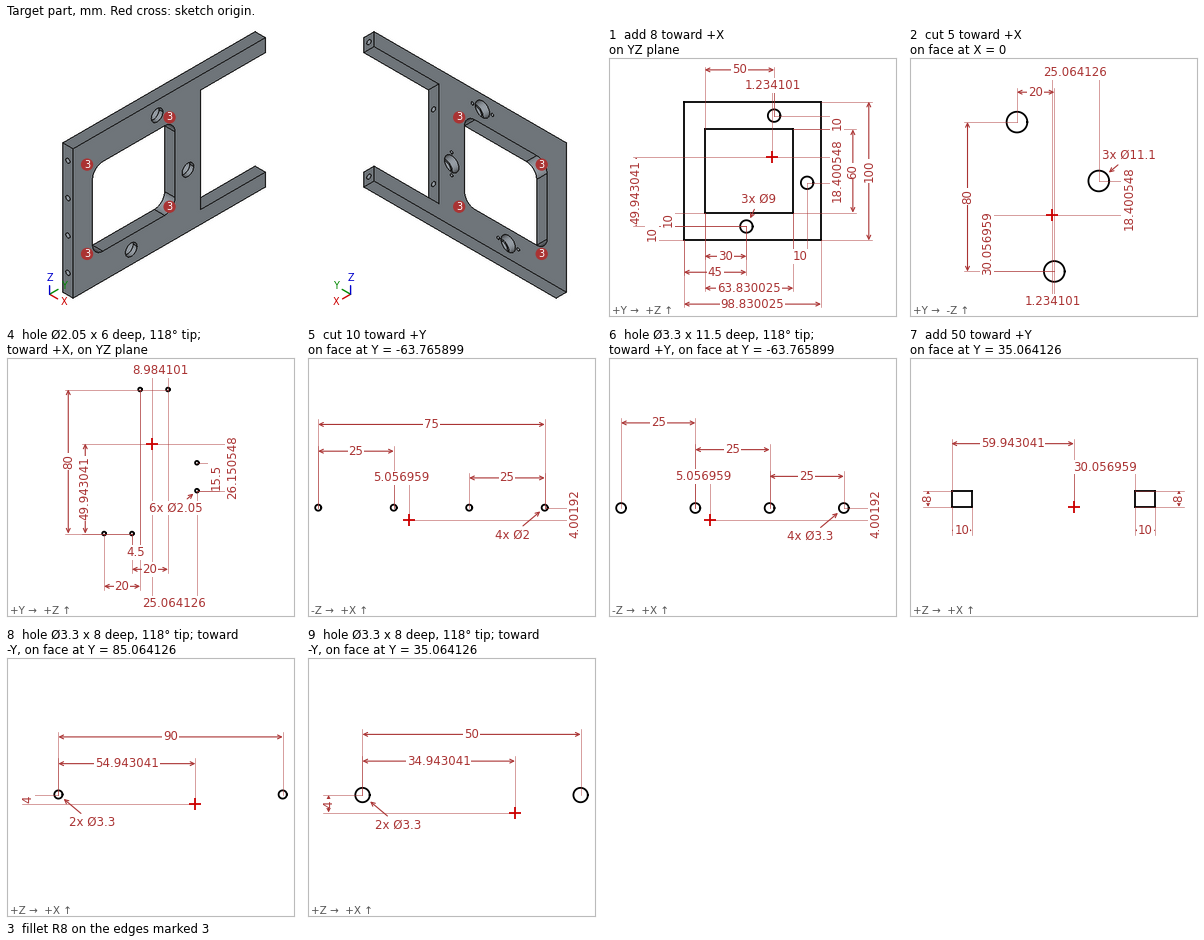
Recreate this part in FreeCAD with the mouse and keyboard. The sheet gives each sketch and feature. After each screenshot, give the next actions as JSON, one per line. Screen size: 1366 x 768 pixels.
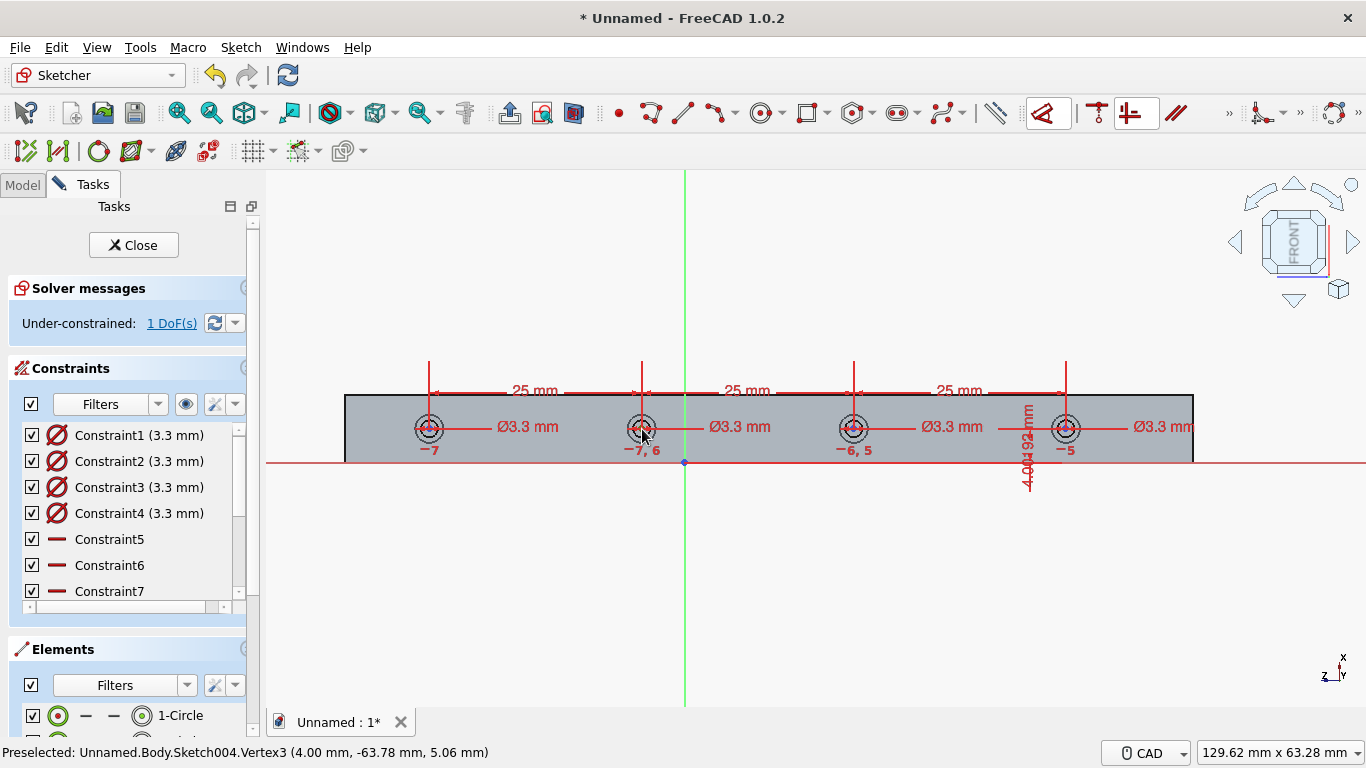
{"action": "left_click", "coordinate": [1066, 114]}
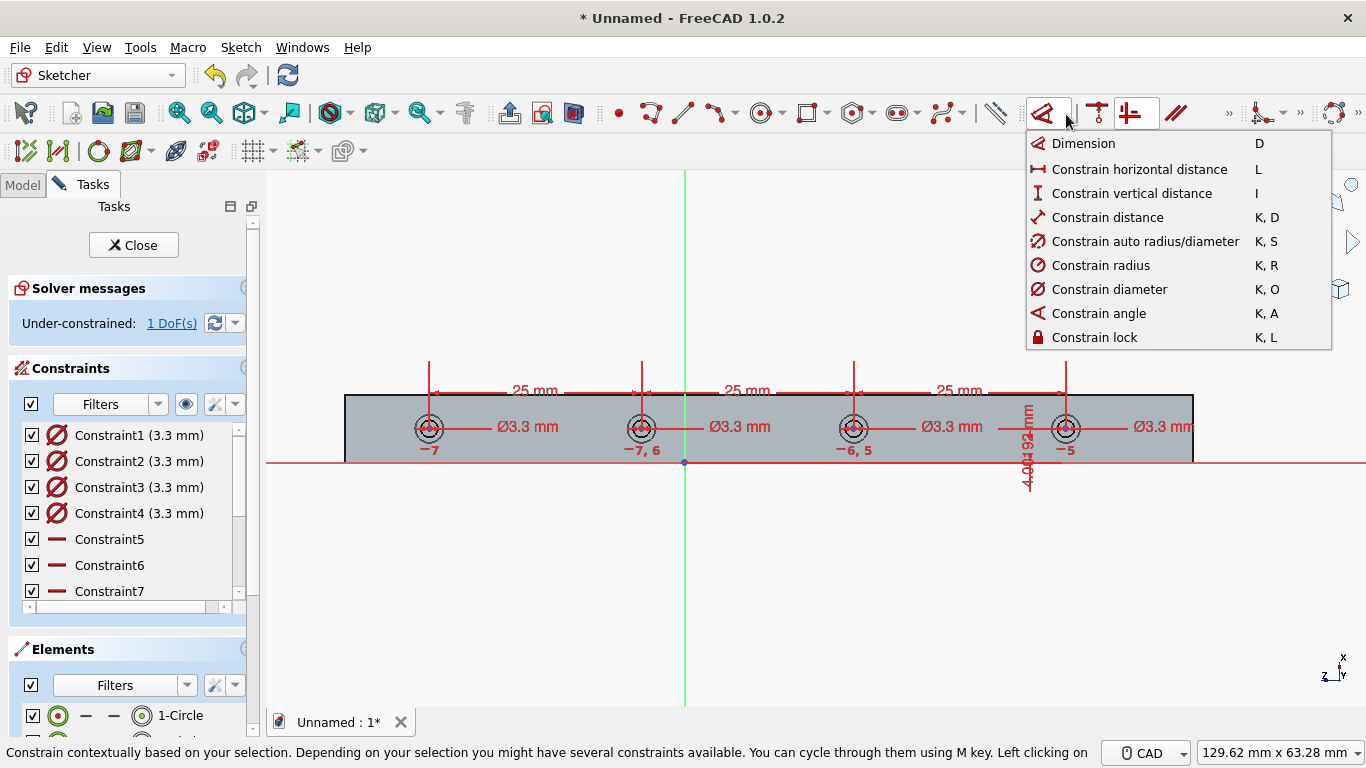
{"action": "left_click", "coordinate": [1179, 169]}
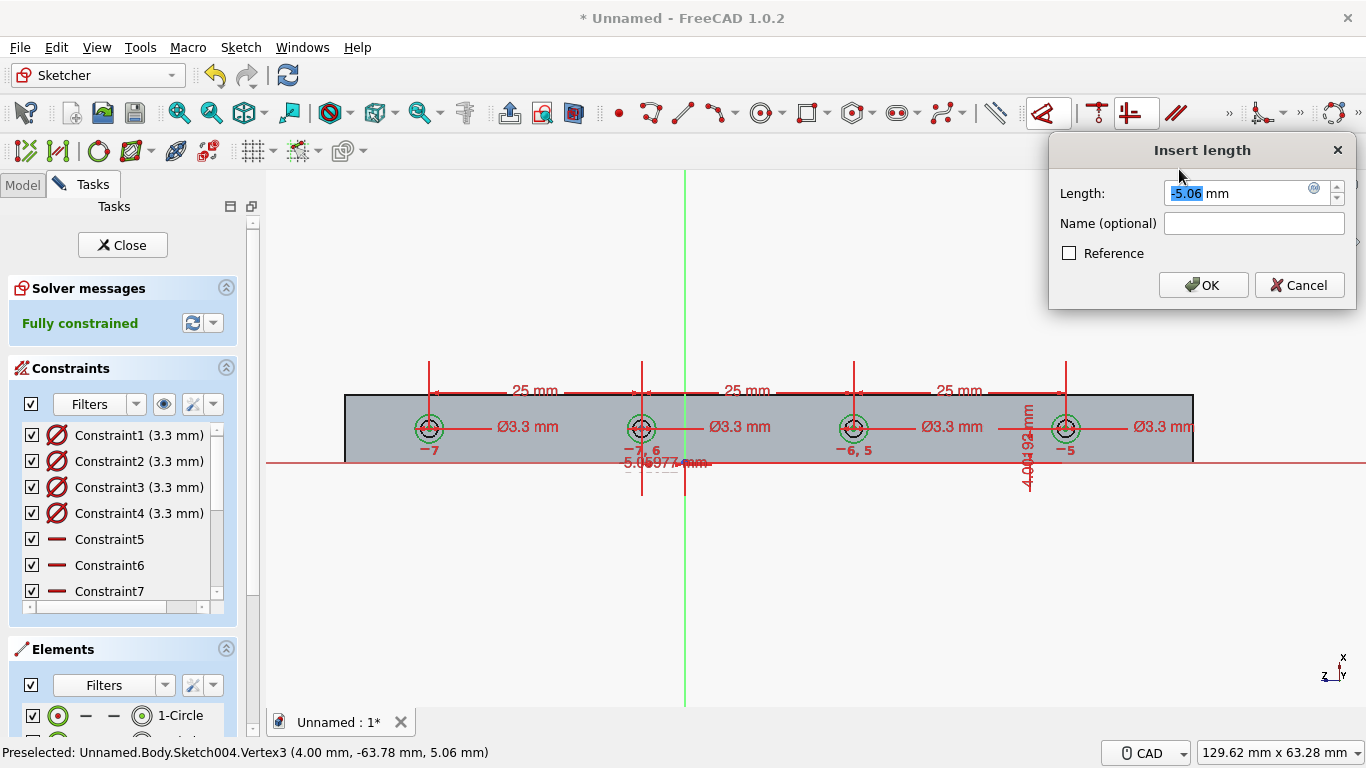
{"action": "type", "text": "-5.056959"}
{"action": "key", "text": "Return"}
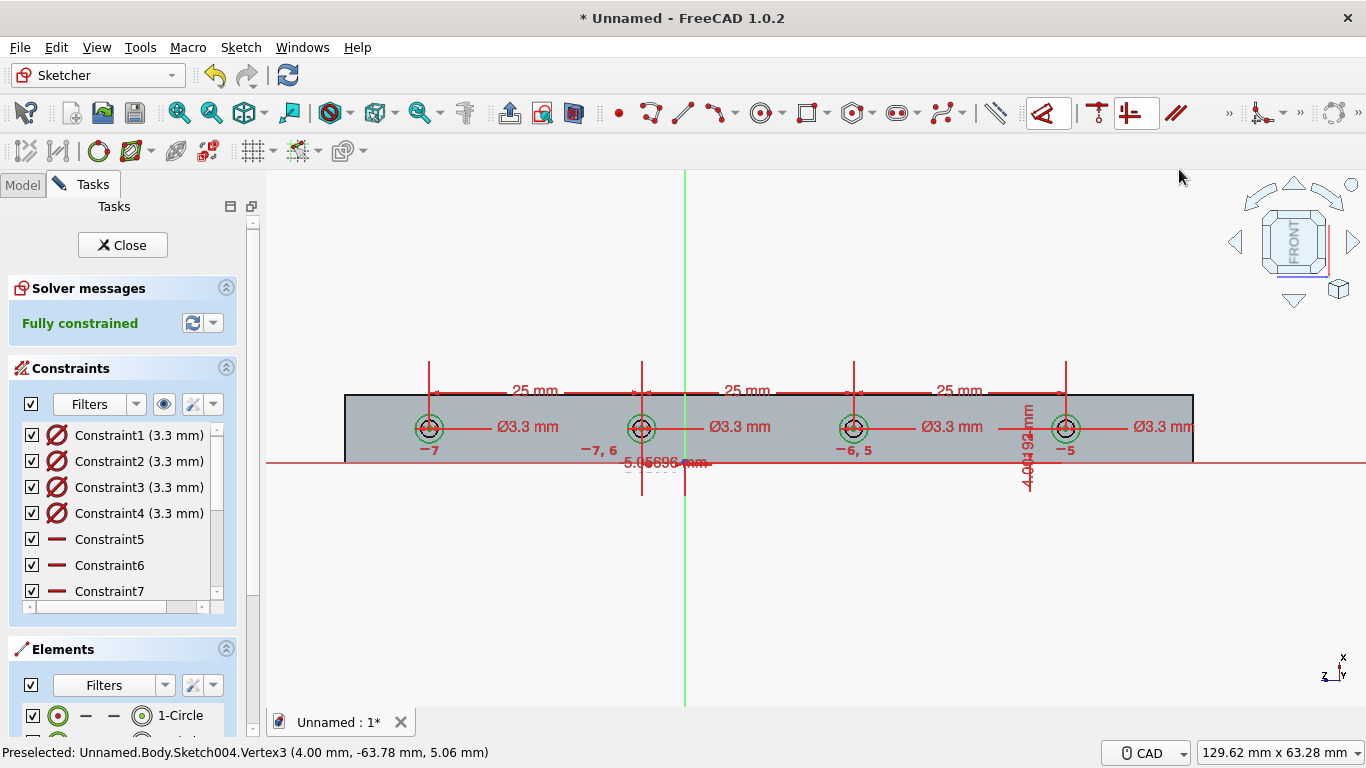
{"action": "left_click", "coordinate": [123, 245]}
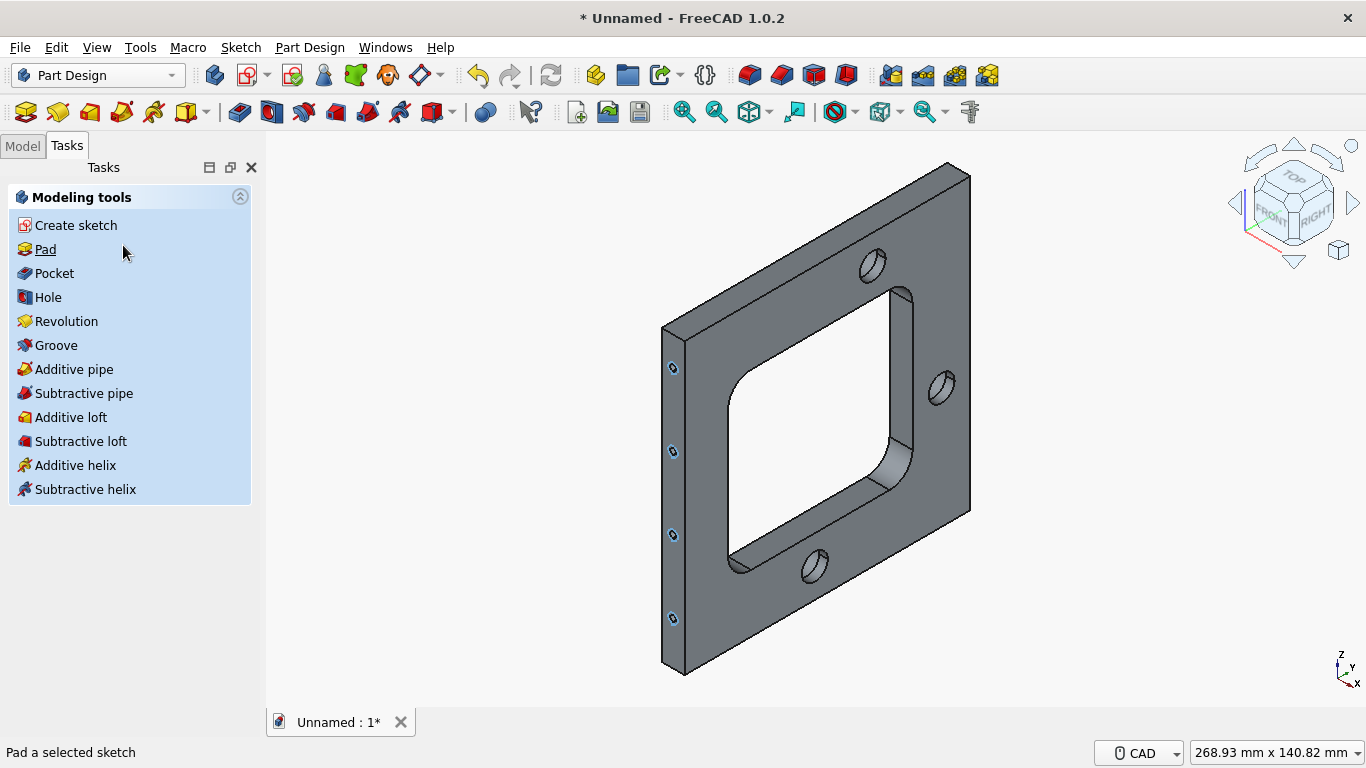
{"action": "left_click", "coordinate": [272, 112]}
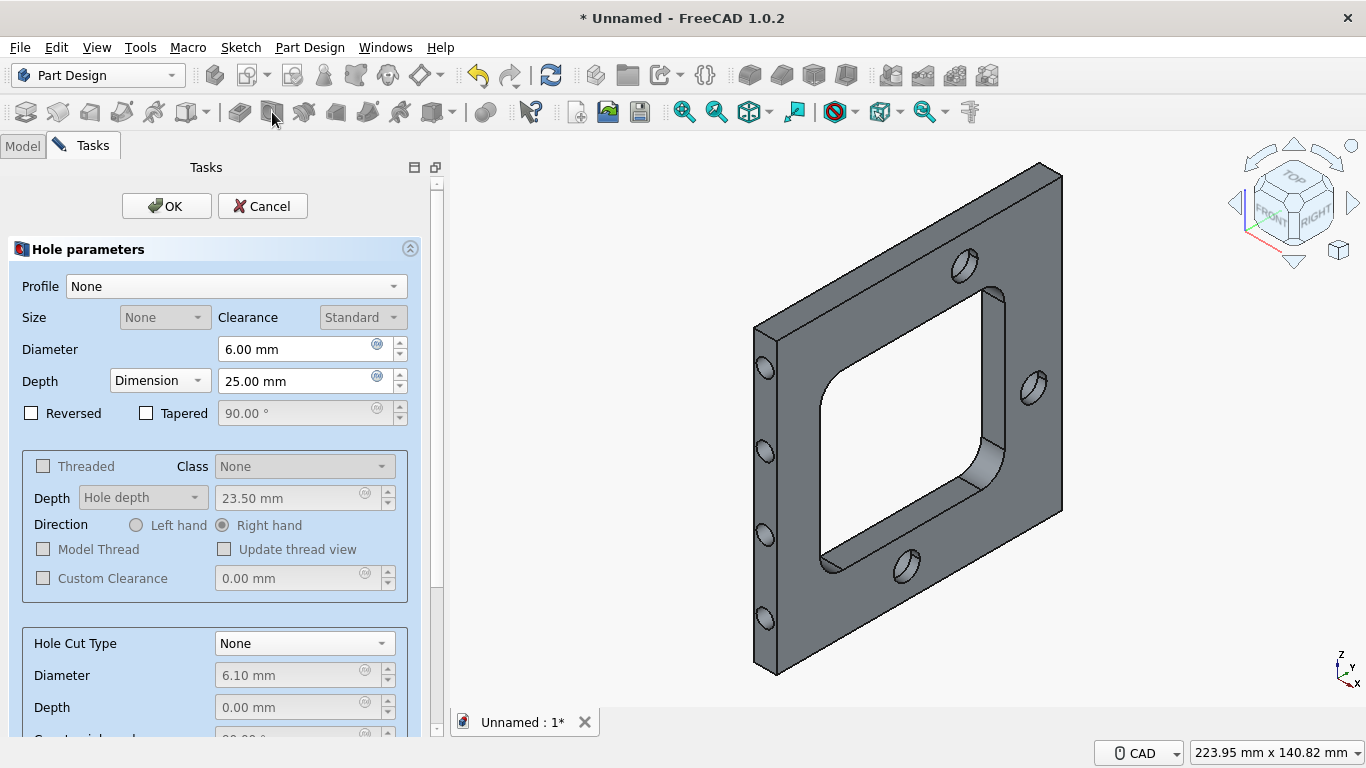
{"action": "triple_click", "coordinate": [305, 349]}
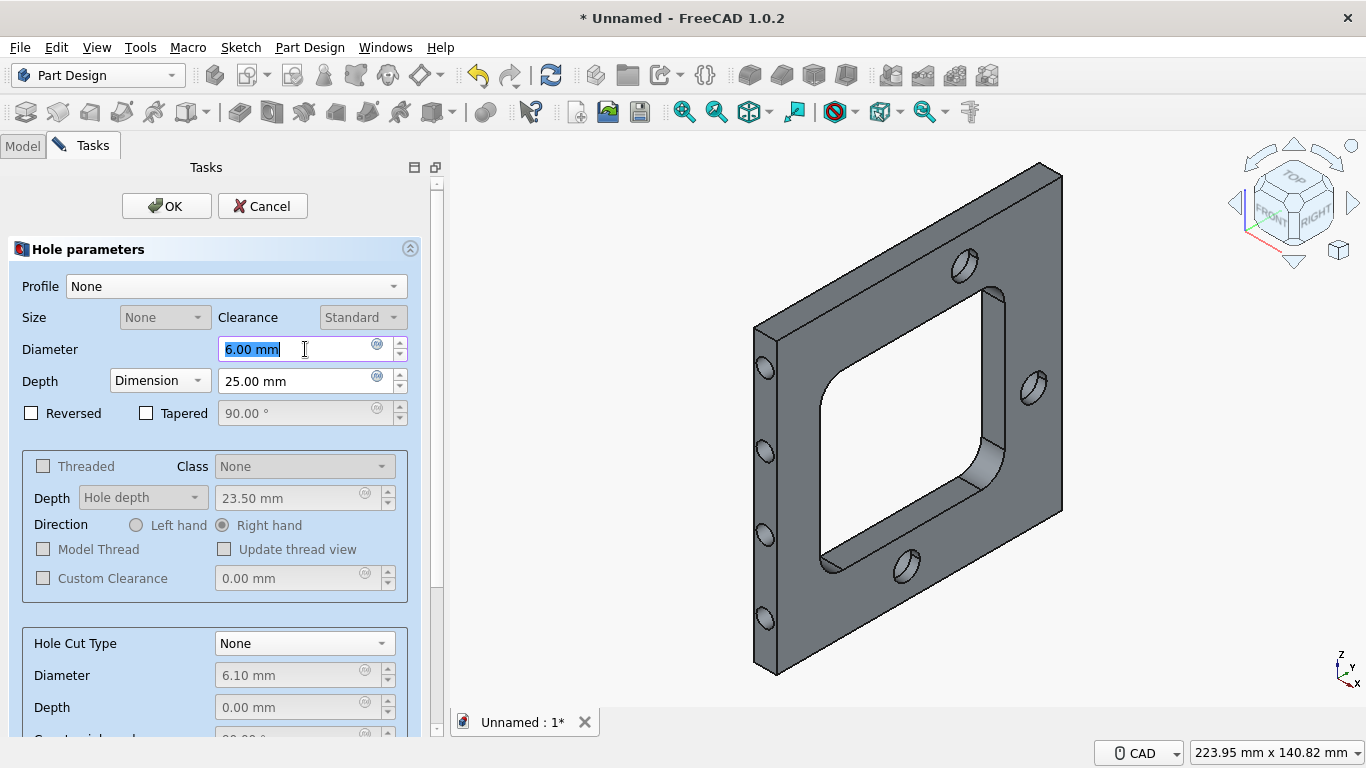
{"action": "type", "text": "3.3"}
{"action": "key", "text": "Tab"}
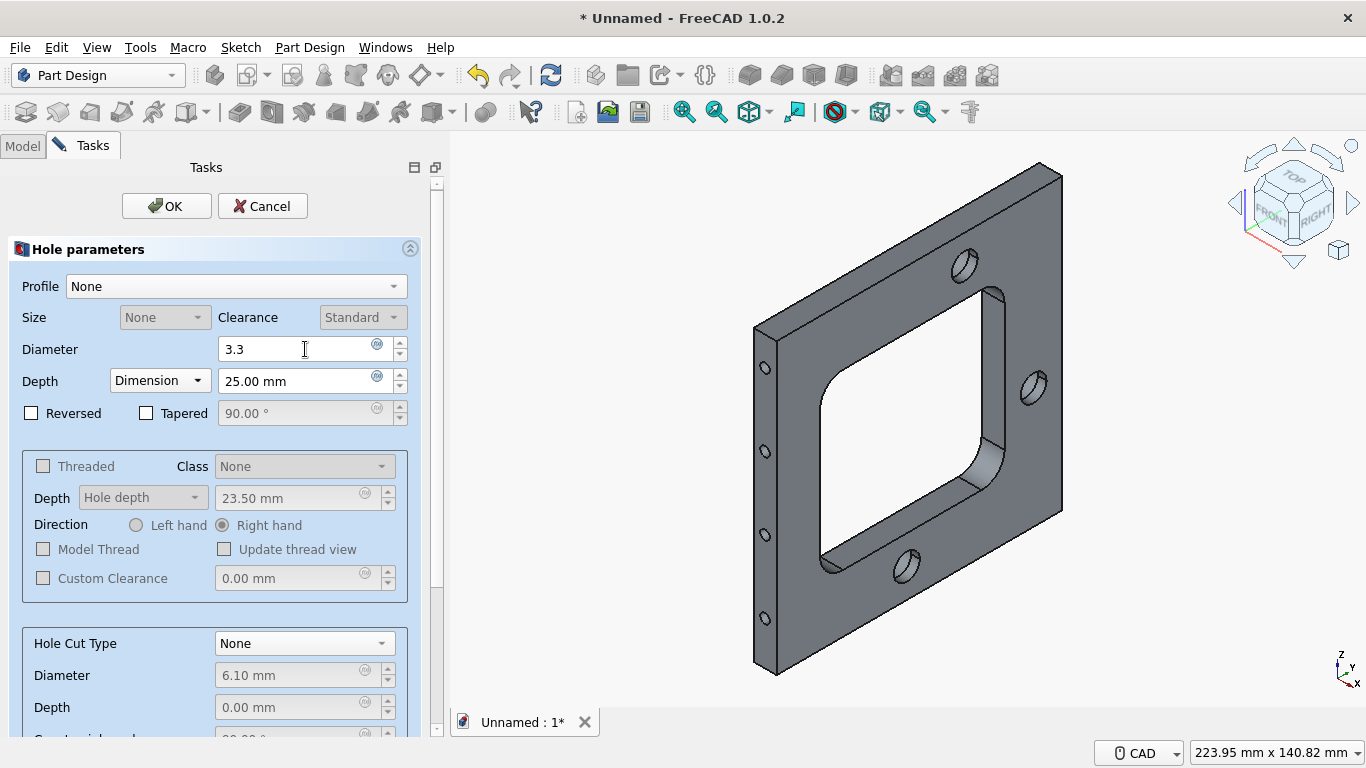
{"action": "triple_click", "coordinate": [305, 381]}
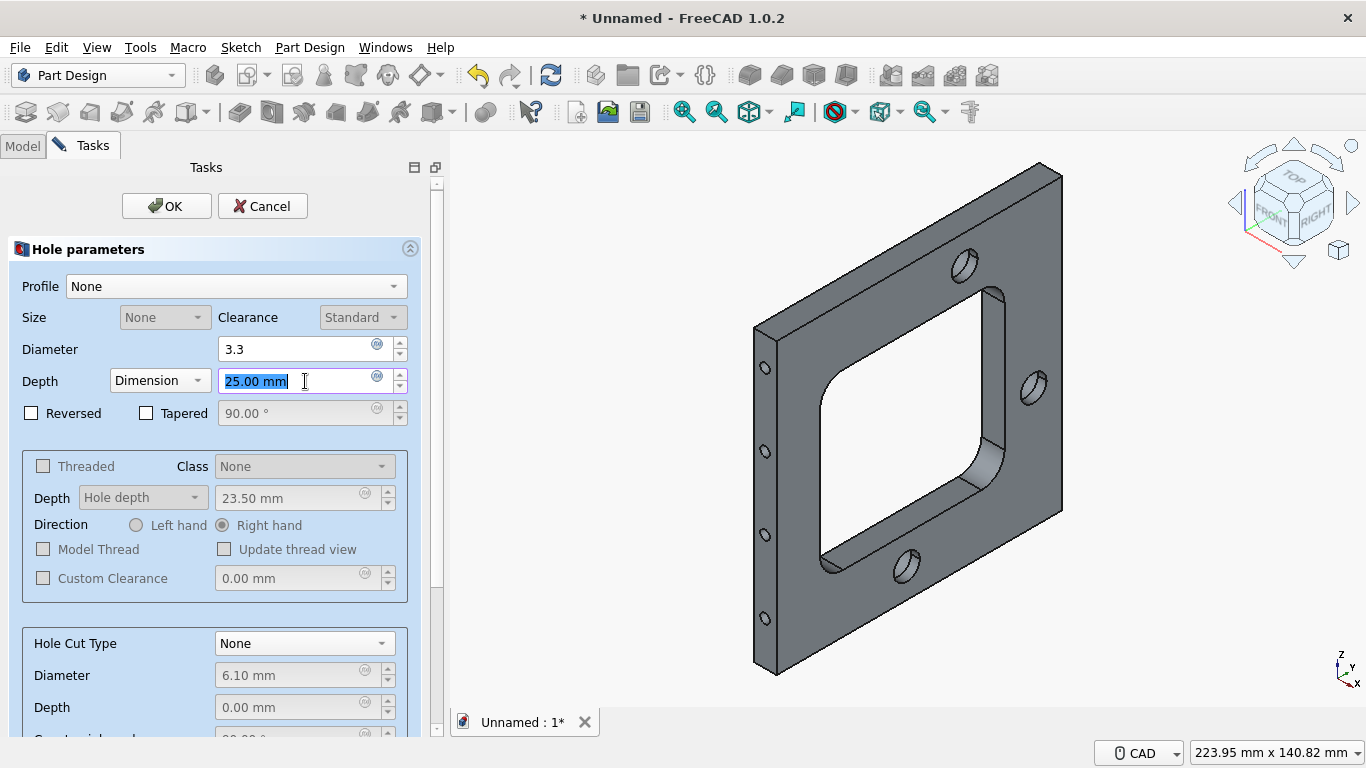
{"action": "type", "text": "11.5"}
{"action": "key", "text": "Tab"}